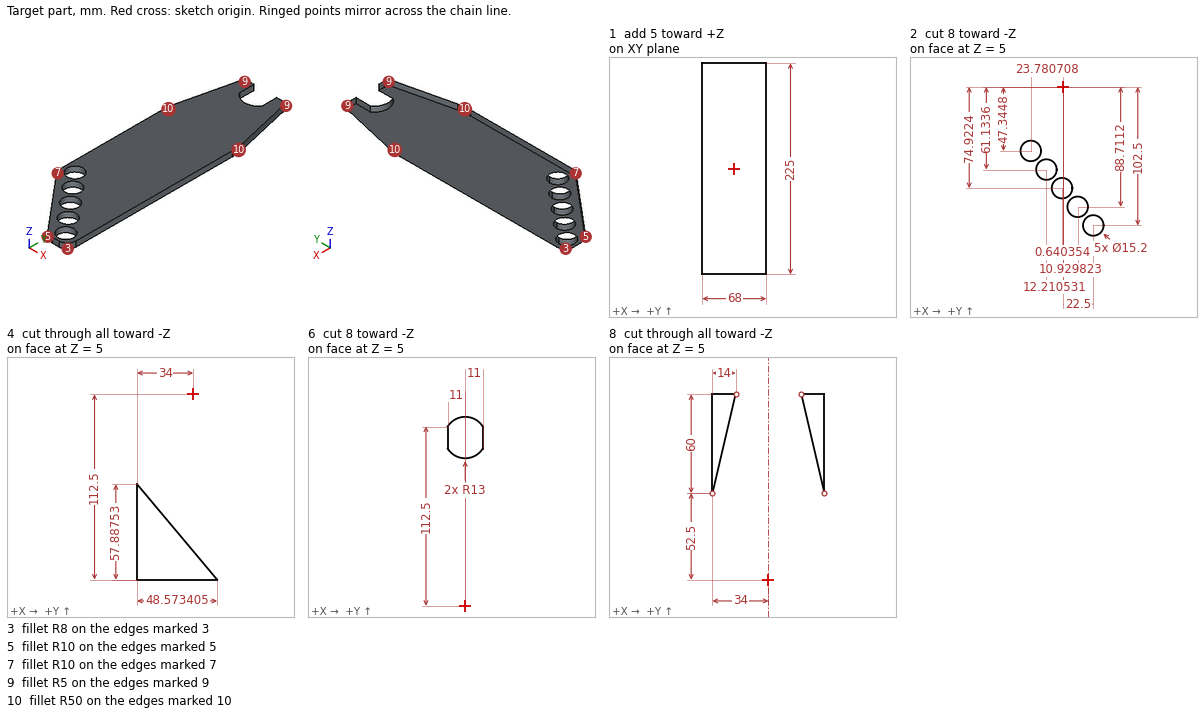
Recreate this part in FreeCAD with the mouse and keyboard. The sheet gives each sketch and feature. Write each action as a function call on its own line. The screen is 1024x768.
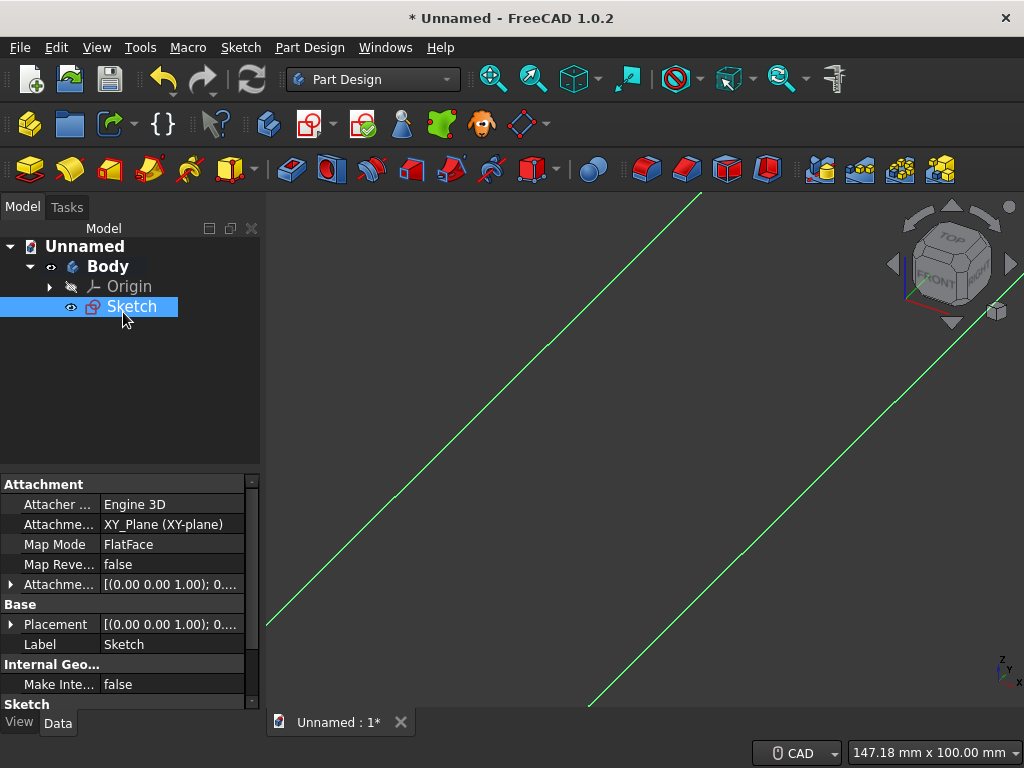
click(30, 170)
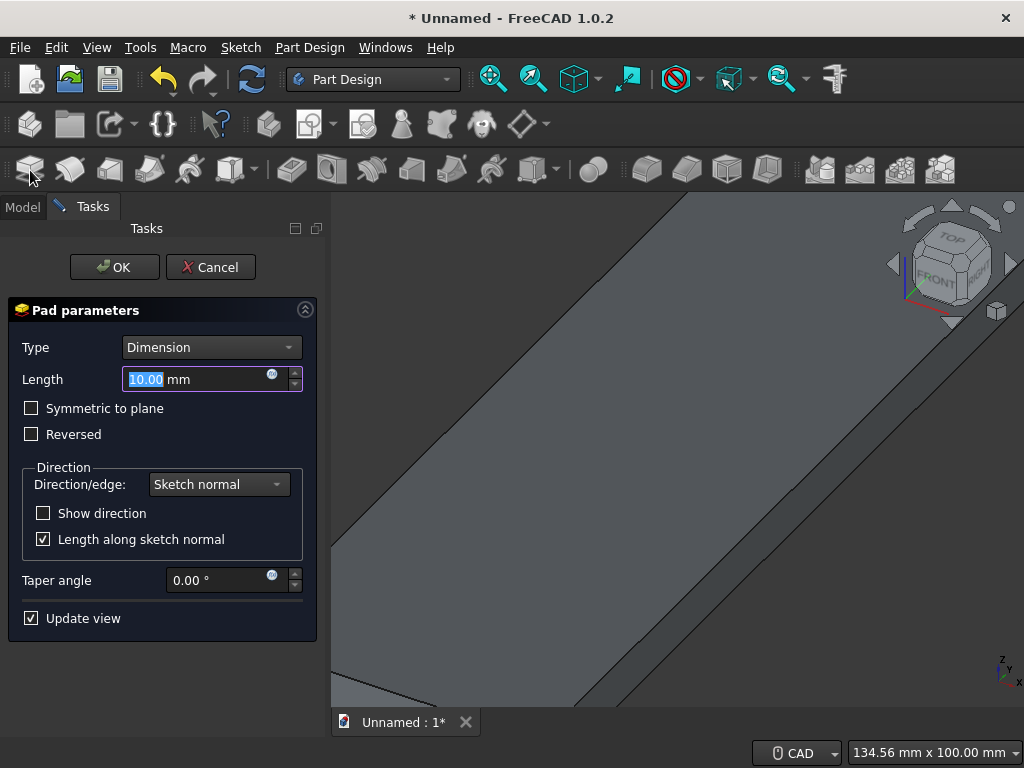
text(5)
key(Tab)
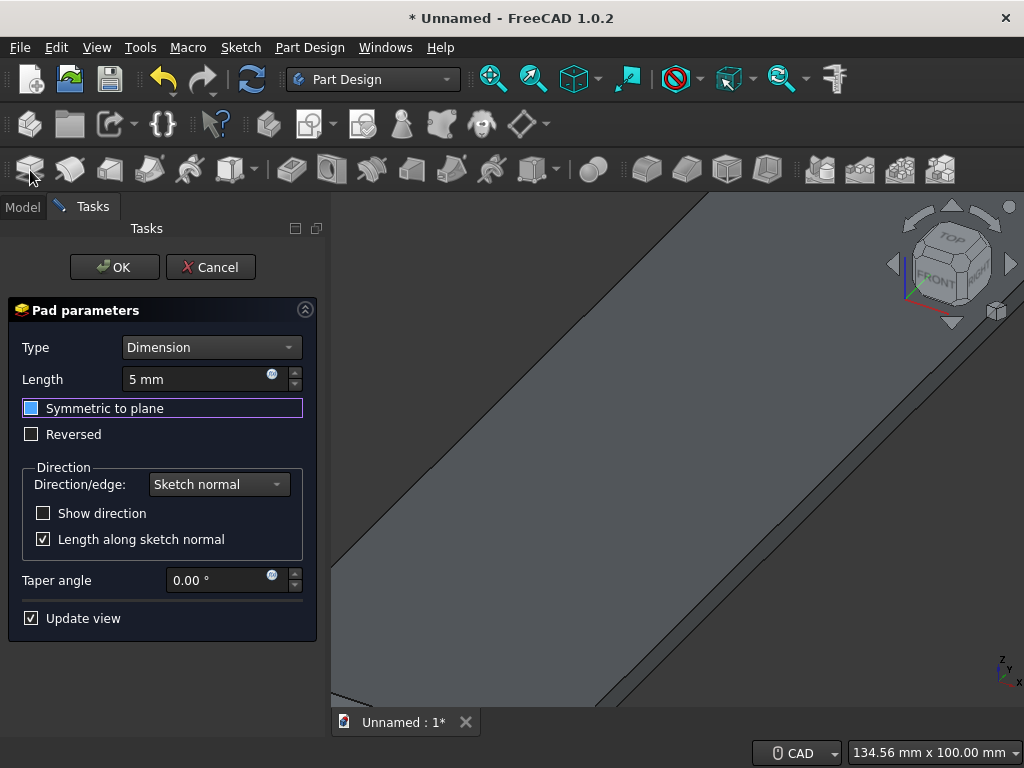
click(115, 267)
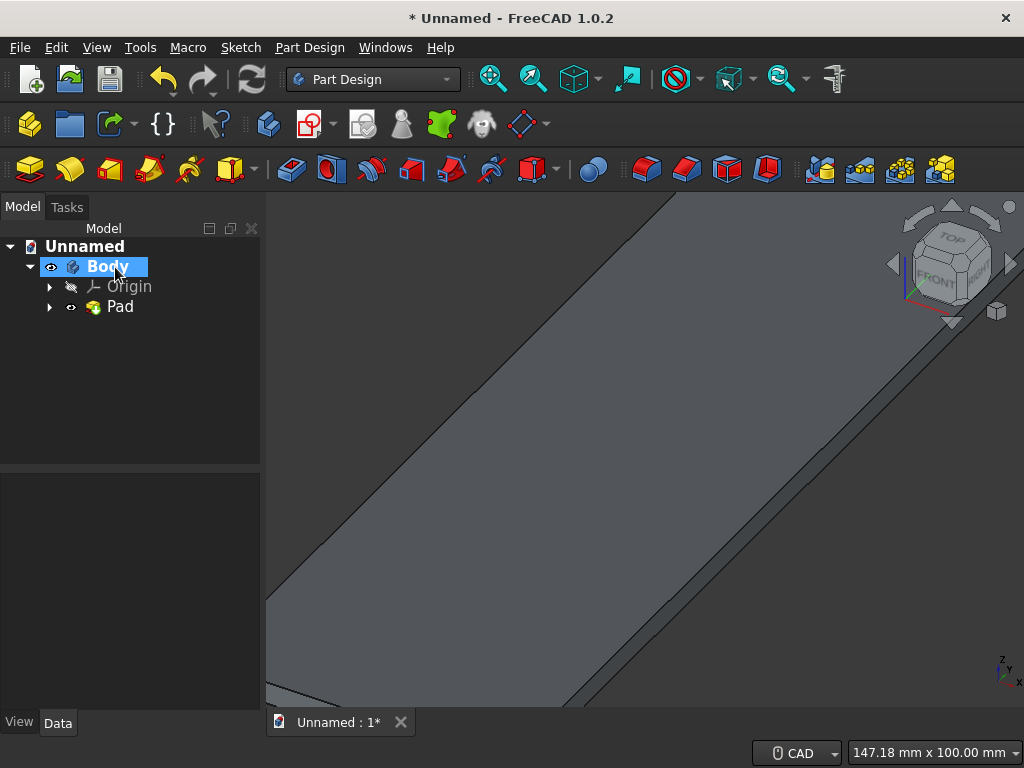
key(v)
key(f)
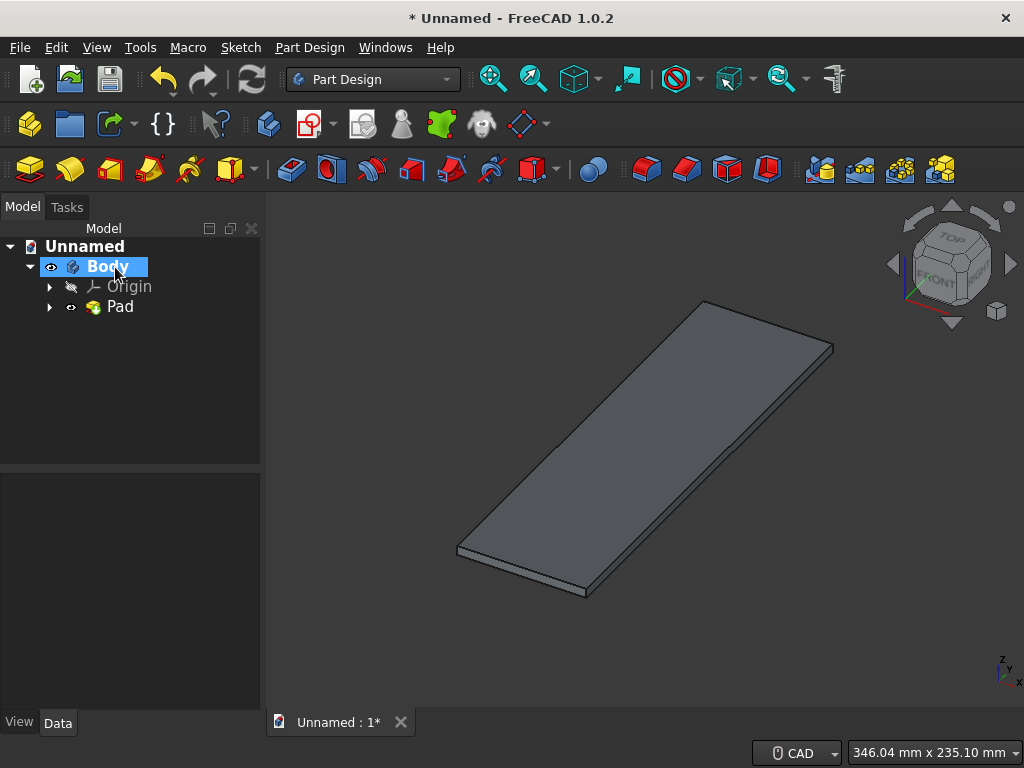
click(715, 374)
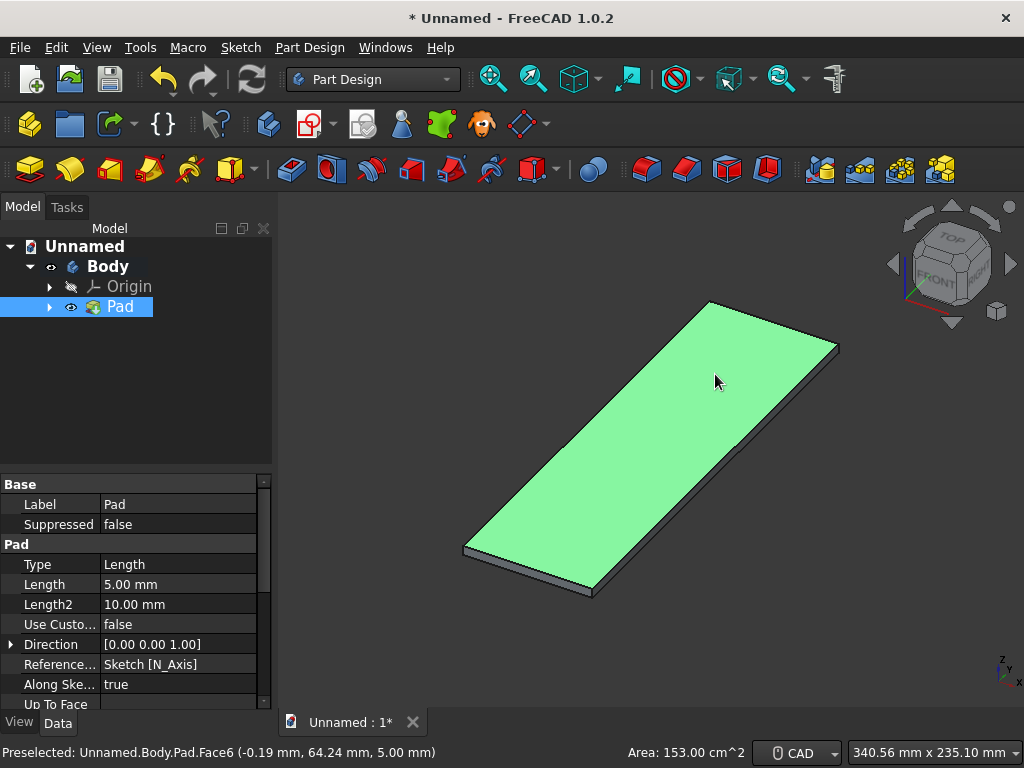
click(310, 124)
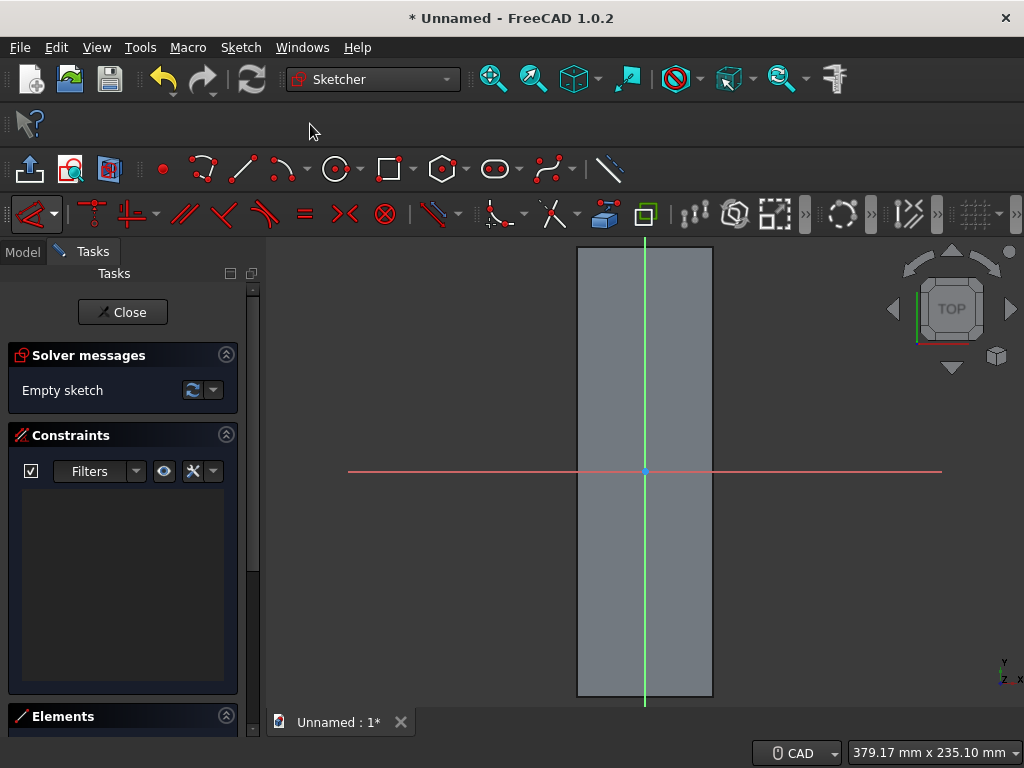
scroll(294, 265, down, 1)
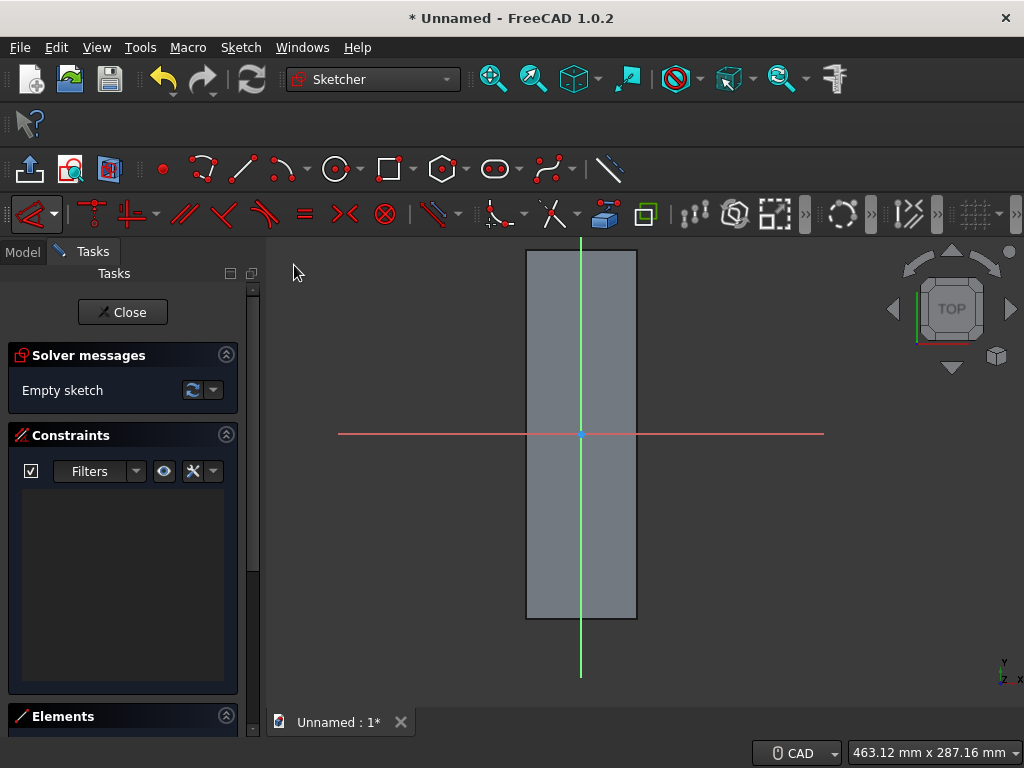
scroll(588, 632, up, 2)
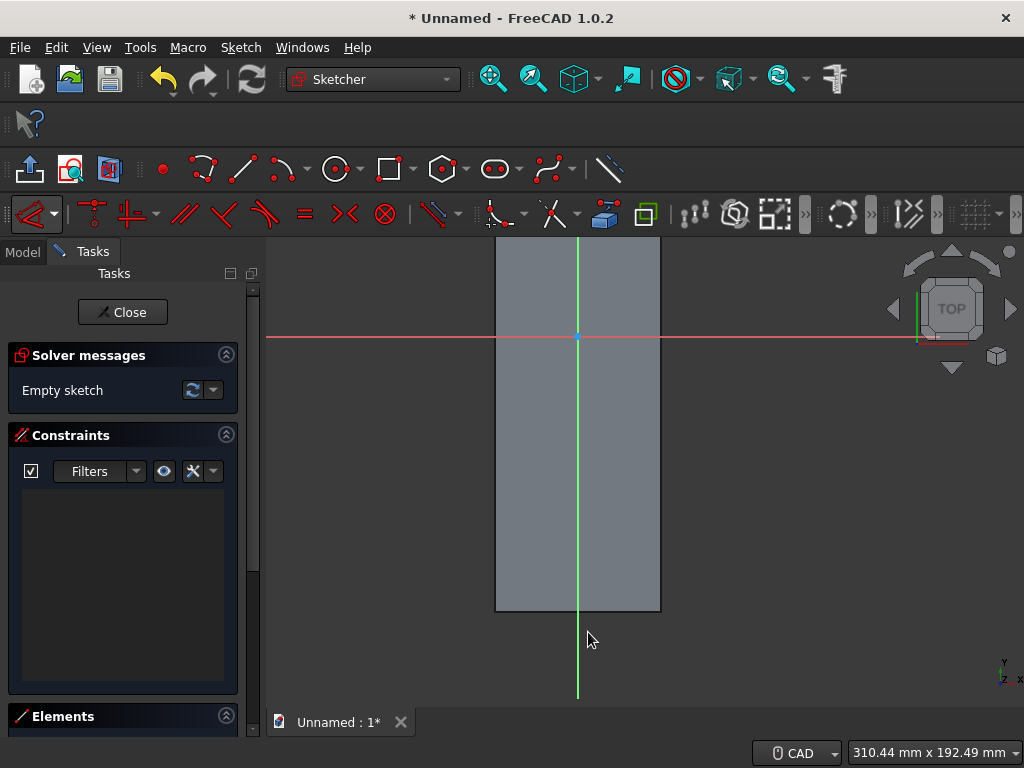
key(g)
key(c)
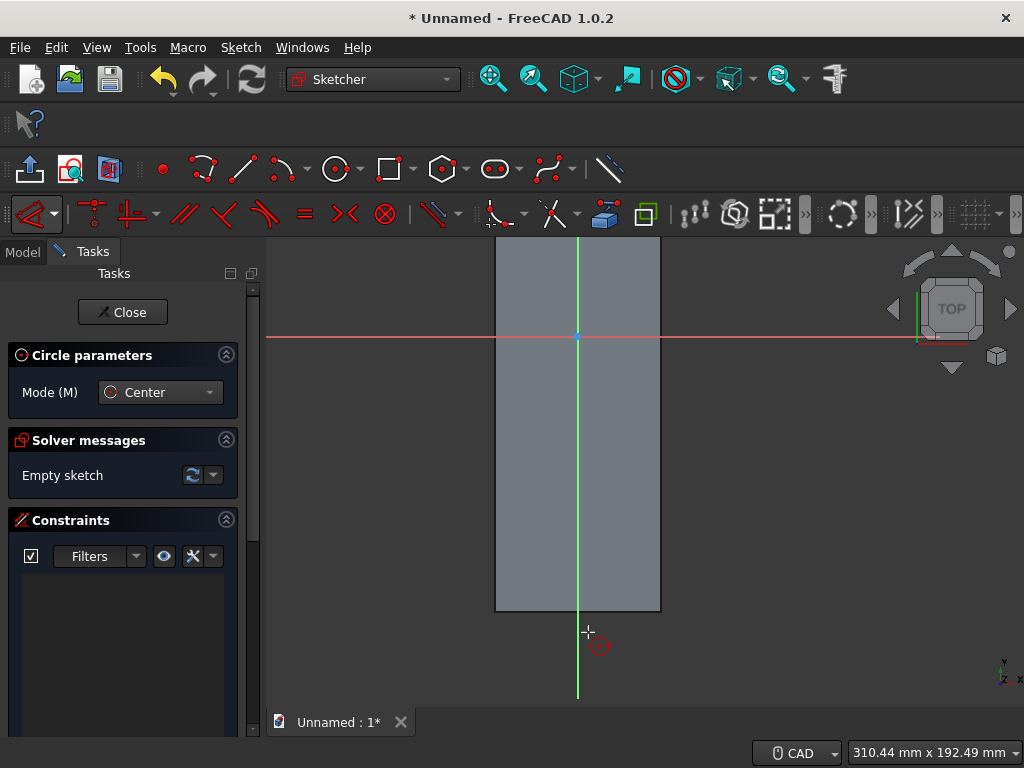
scroll(633, 587, up, 2)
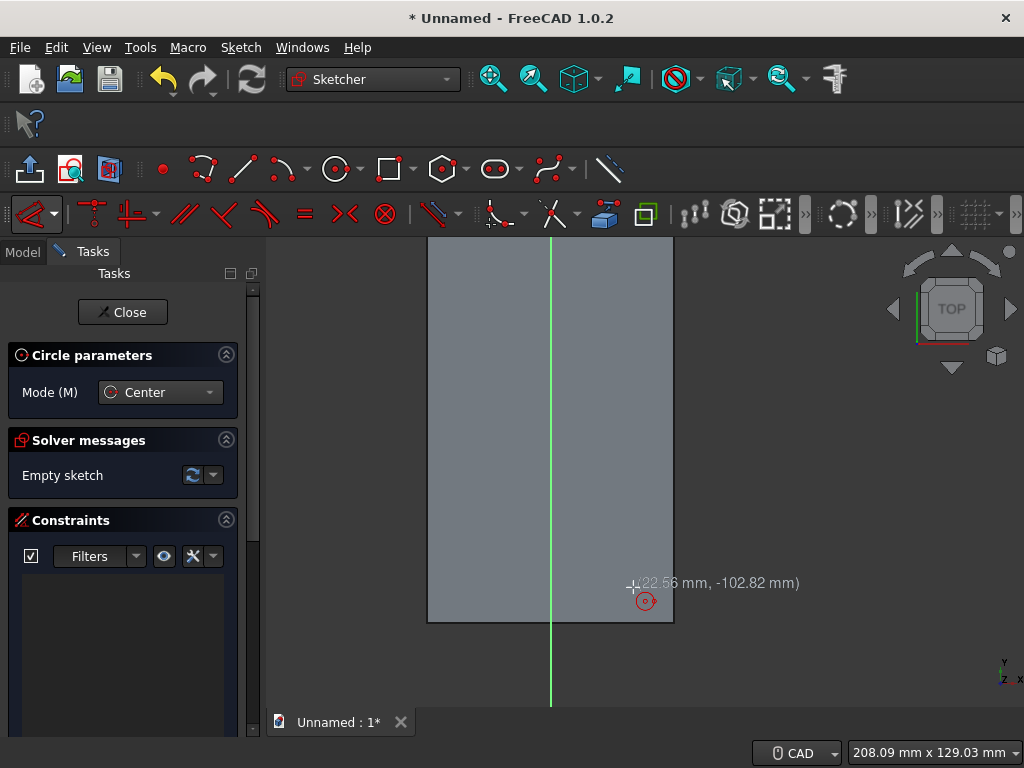
click(633, 587)
click(652, 567)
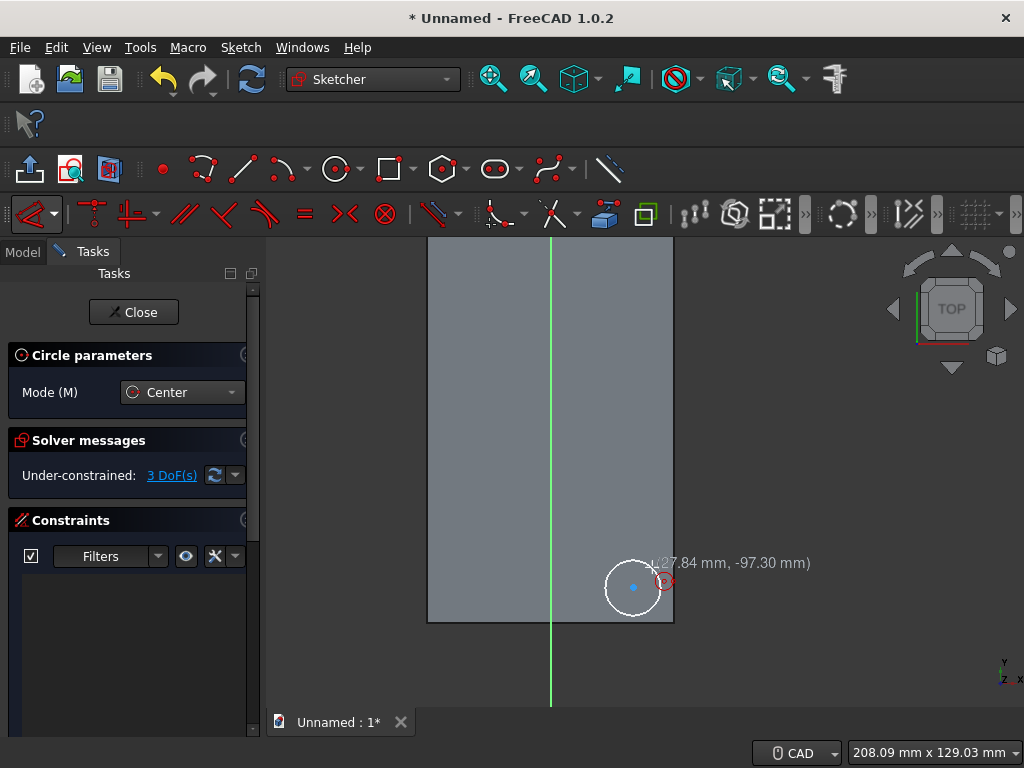
click(590, 537)
click(610, 517)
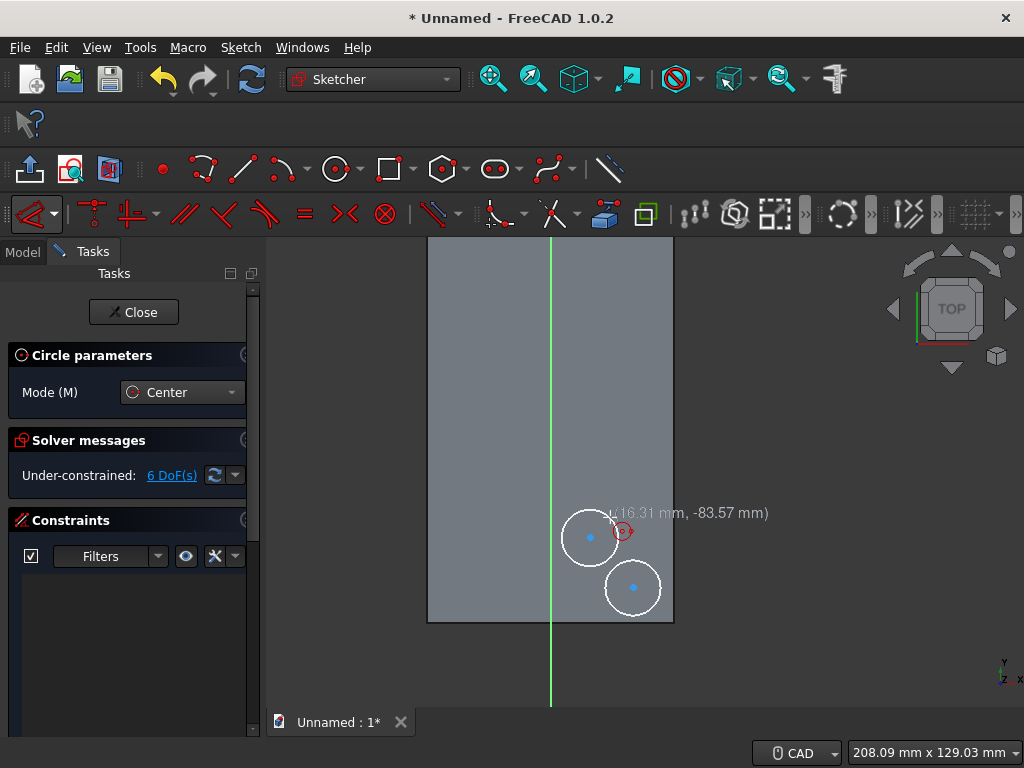
scroll(548, 486, up, 10)